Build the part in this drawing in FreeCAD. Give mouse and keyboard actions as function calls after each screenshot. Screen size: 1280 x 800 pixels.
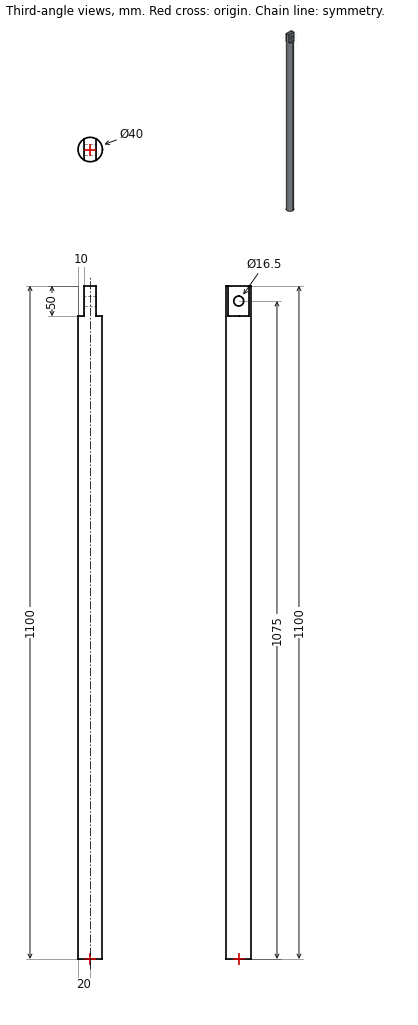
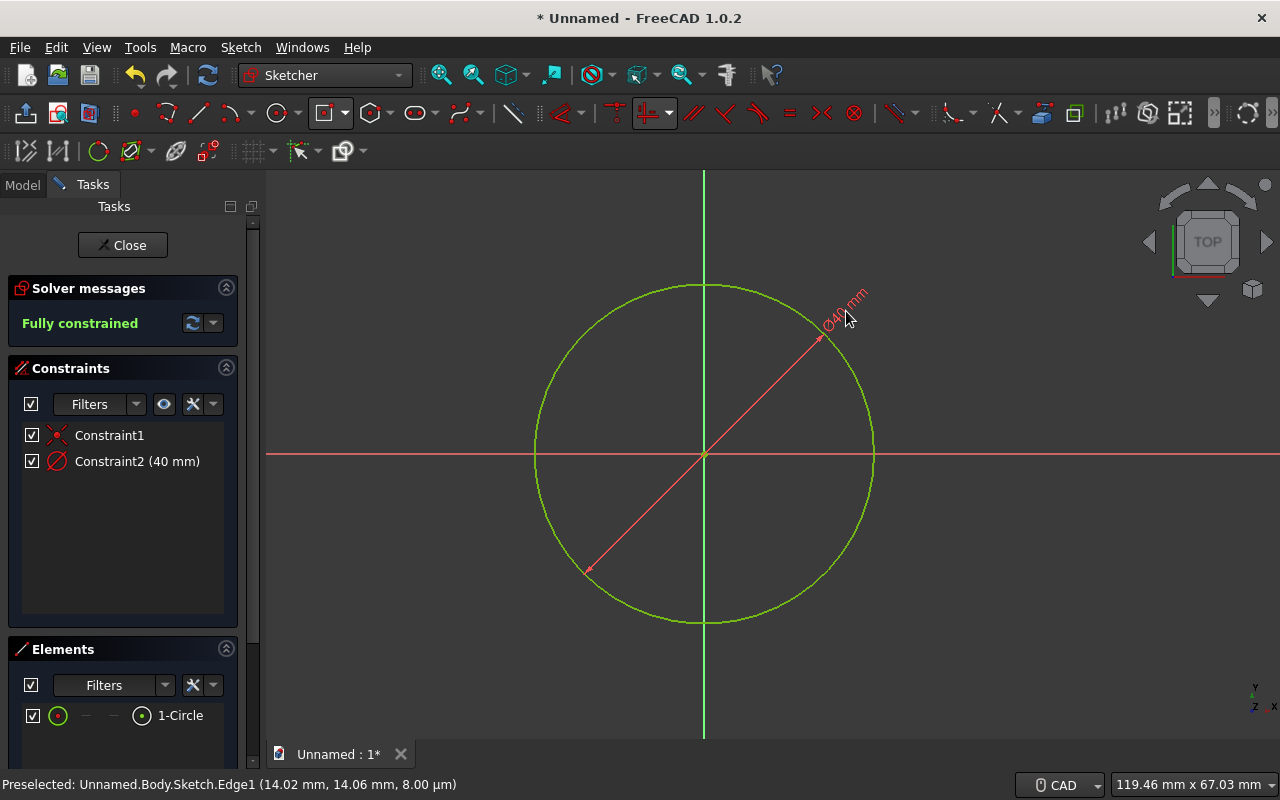
click(123, 245)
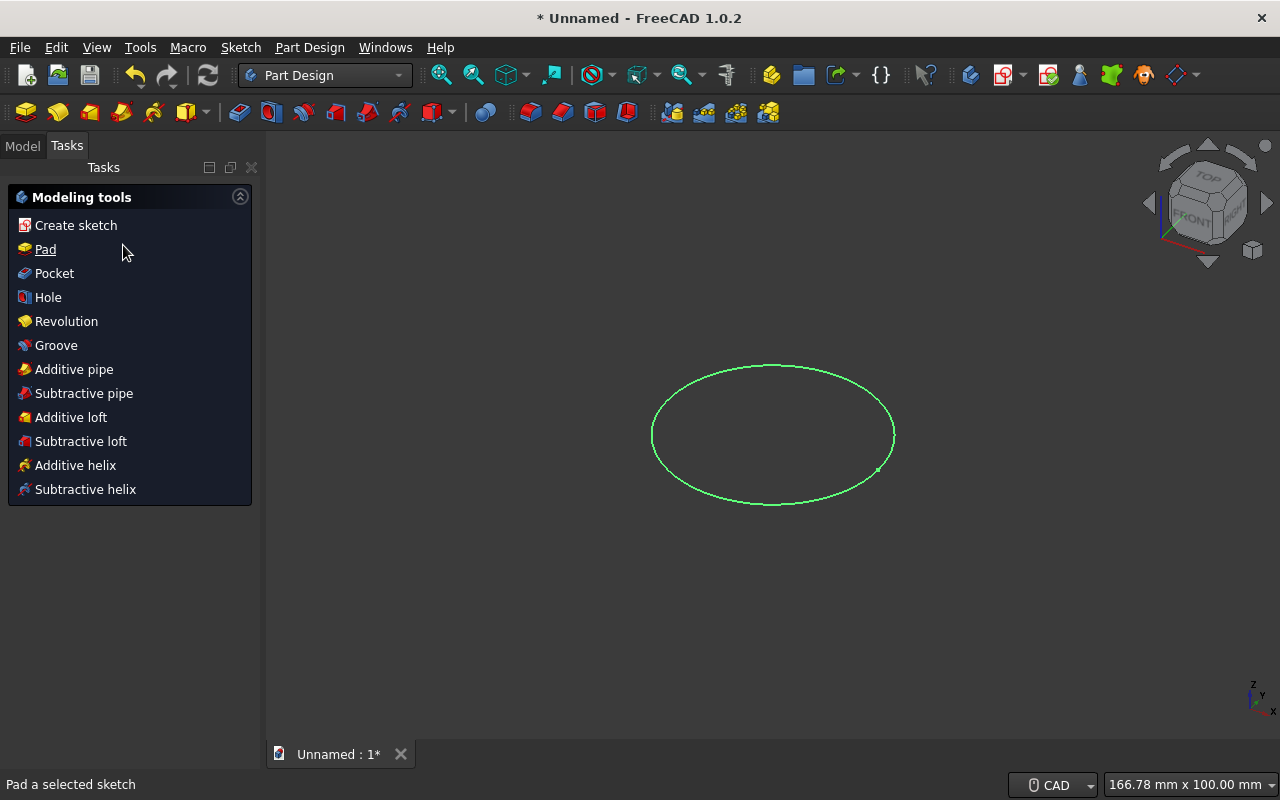
click(26, 112)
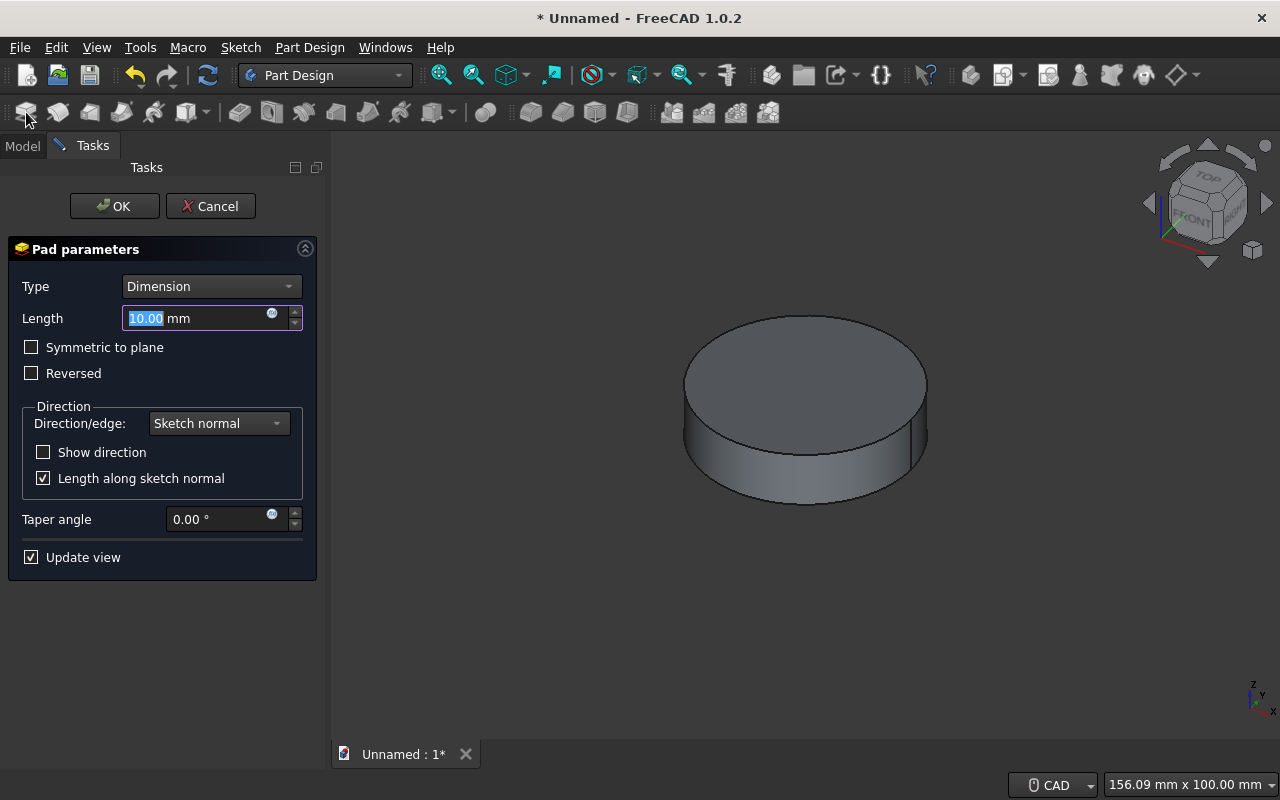
text(1100)
key(Tab)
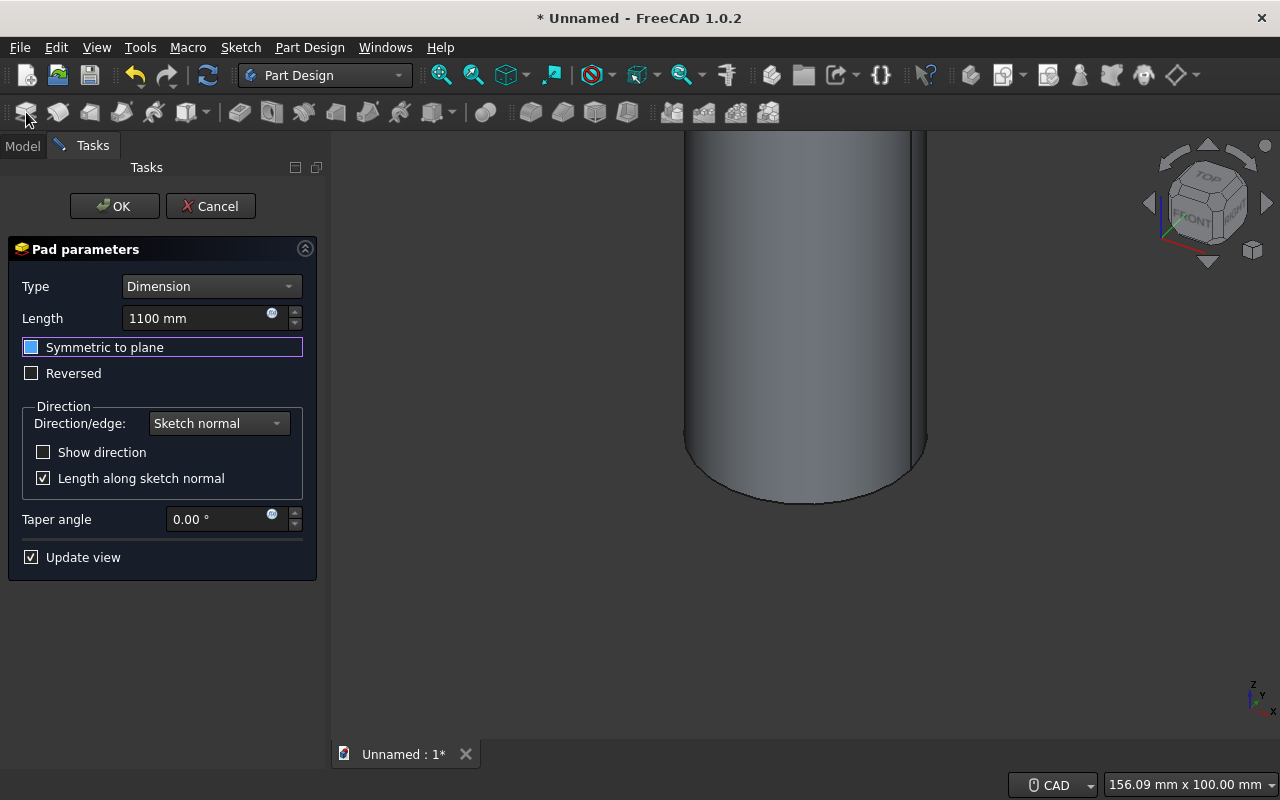
click(115, 206)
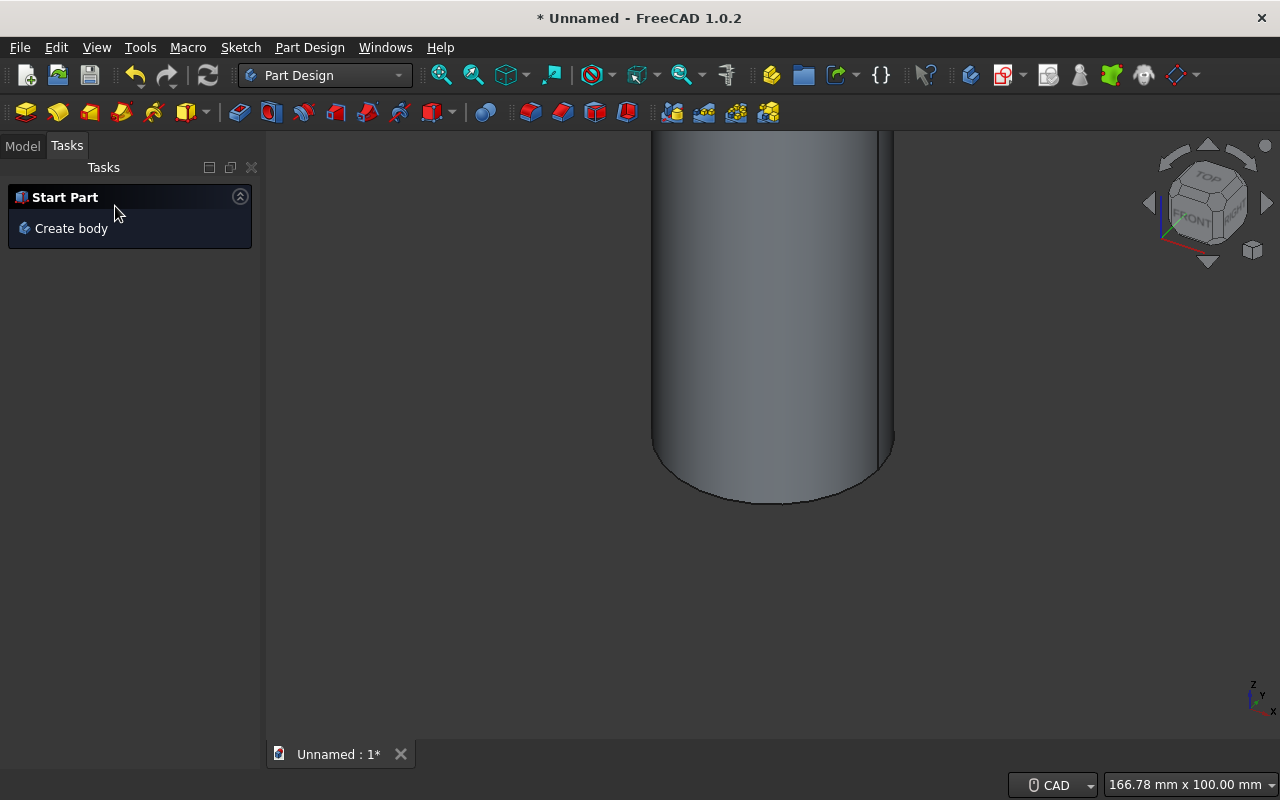
click(442, 76)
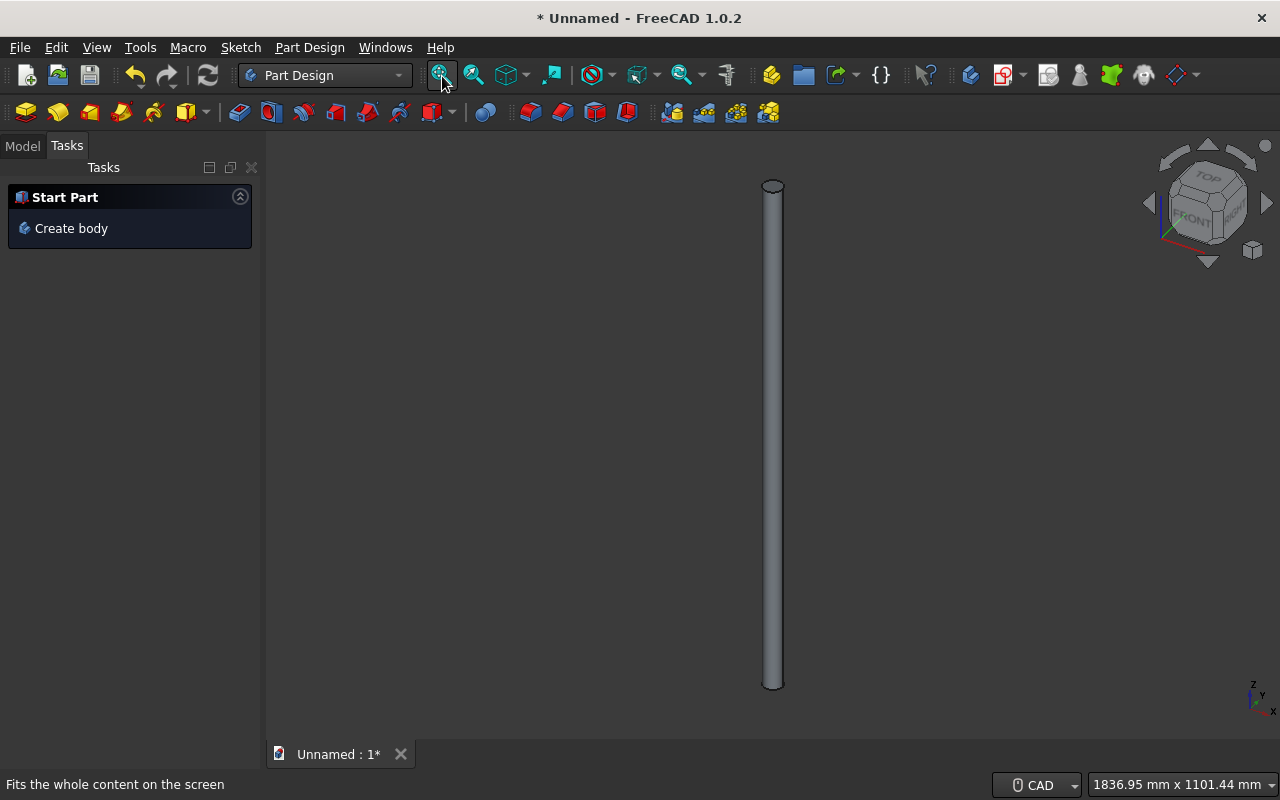
click(1004, 76)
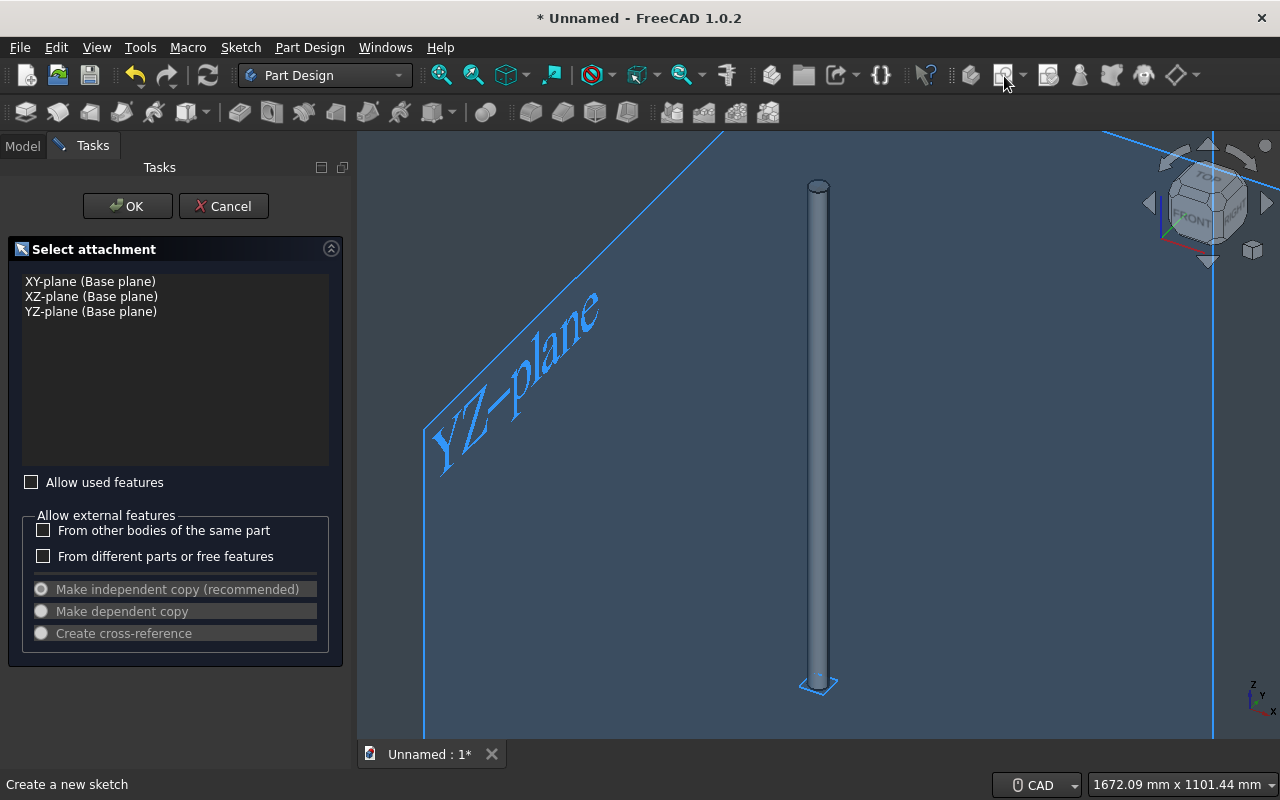
click(82, 296)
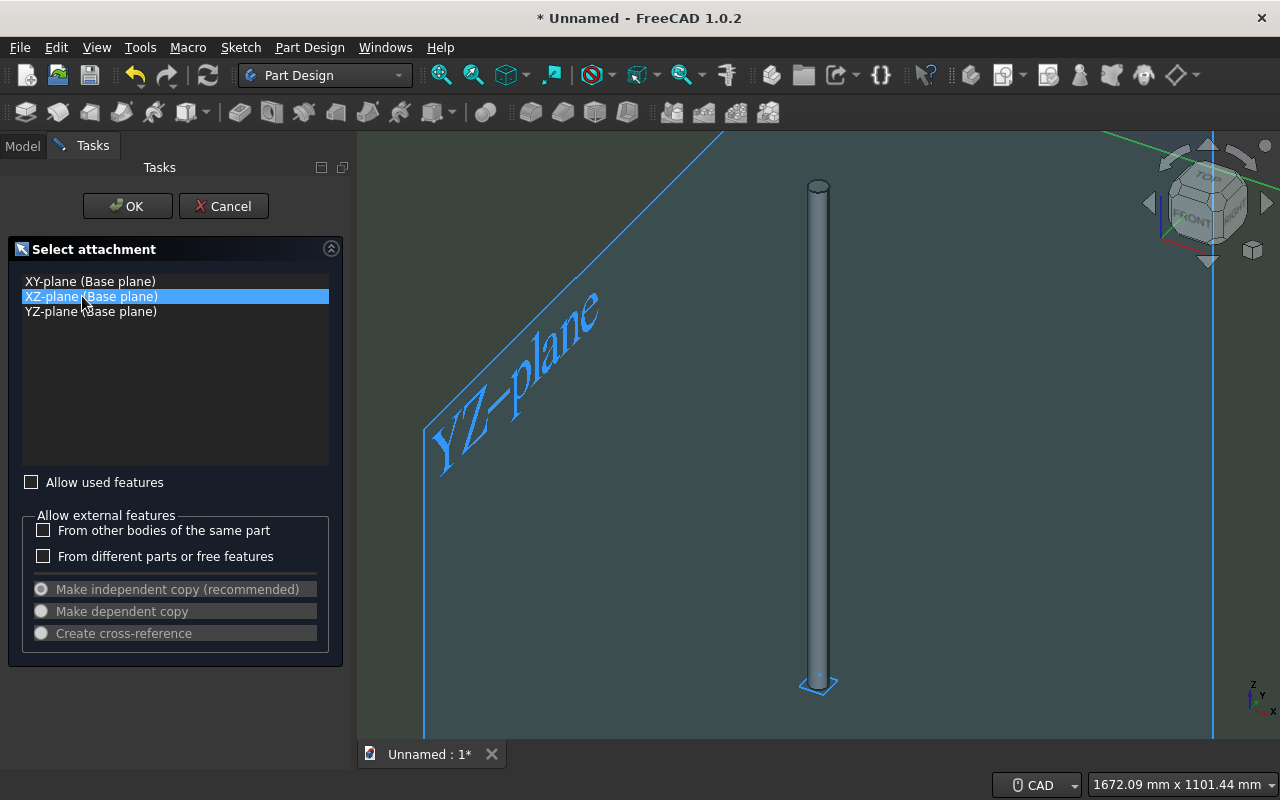
click(128, 206)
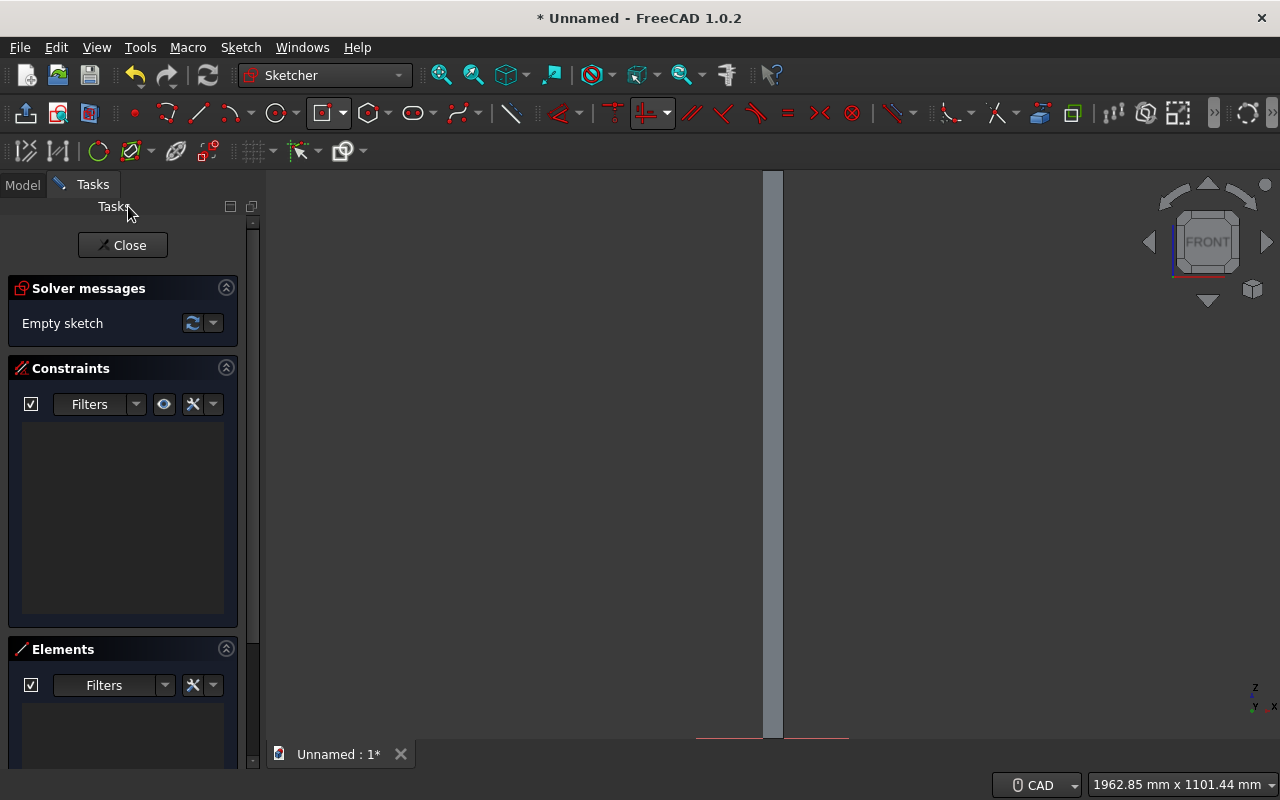
click(90, 114)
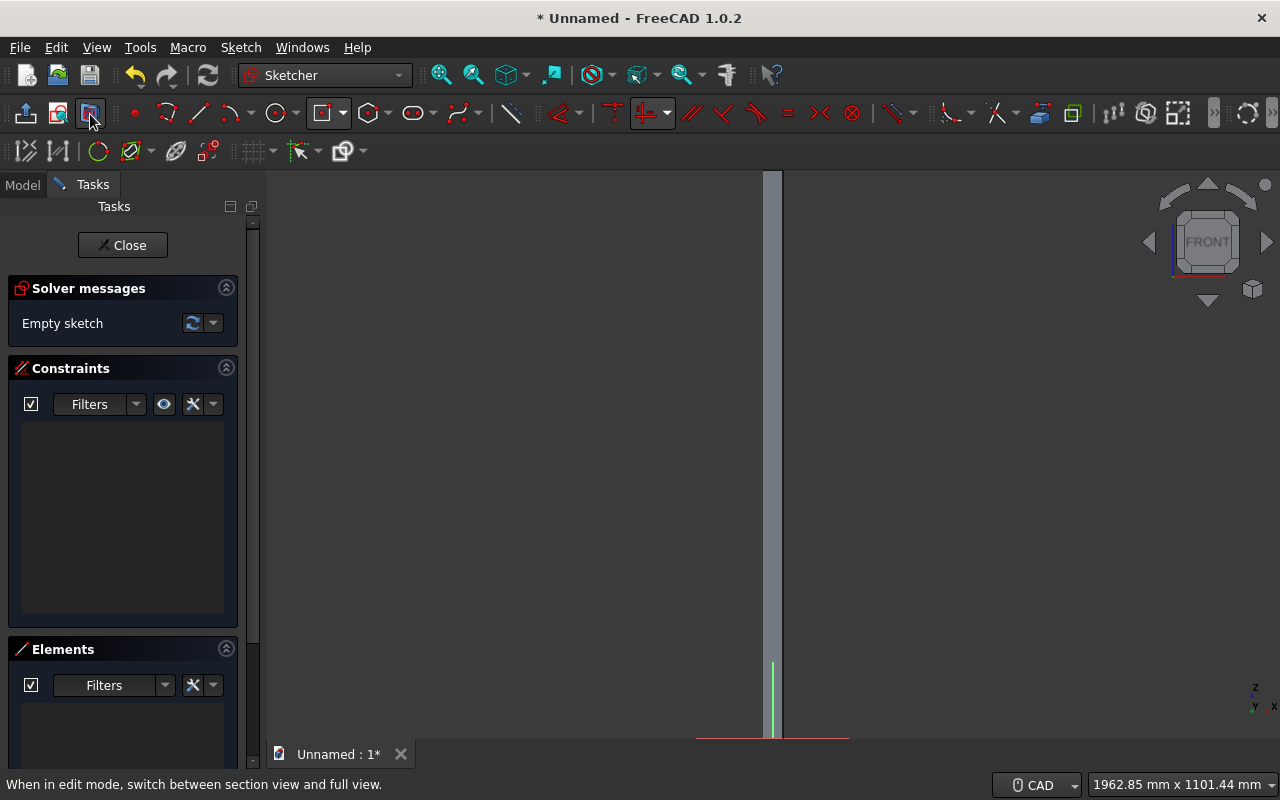
scroll(704, 454, down, 5)